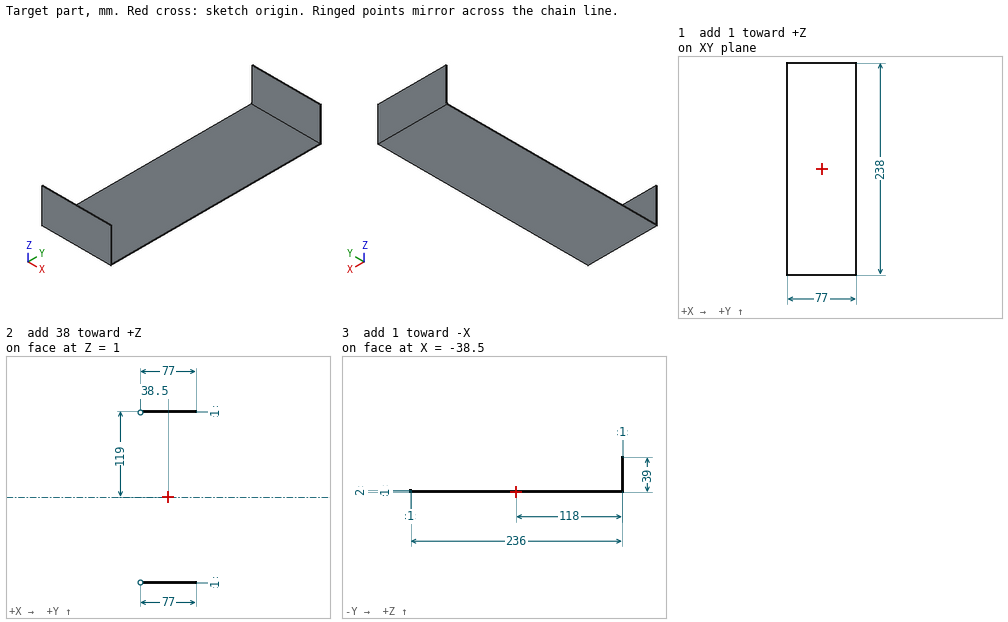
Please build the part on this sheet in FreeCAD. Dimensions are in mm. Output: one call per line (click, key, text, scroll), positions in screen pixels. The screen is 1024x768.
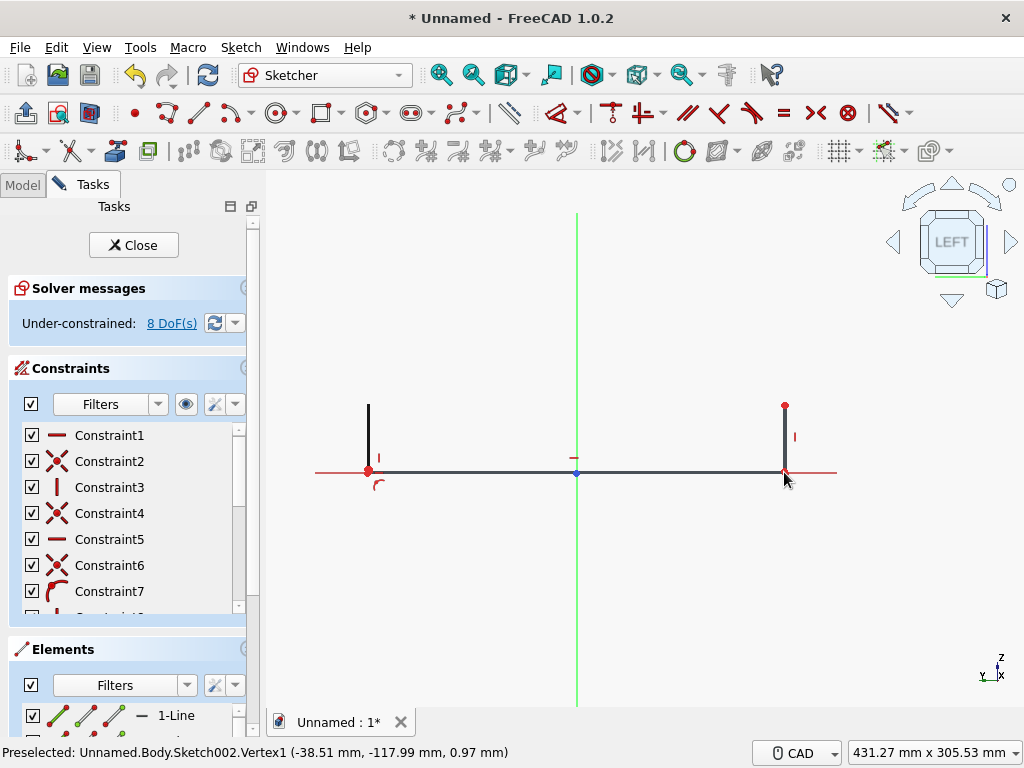
scroll(785, 406, up, 14)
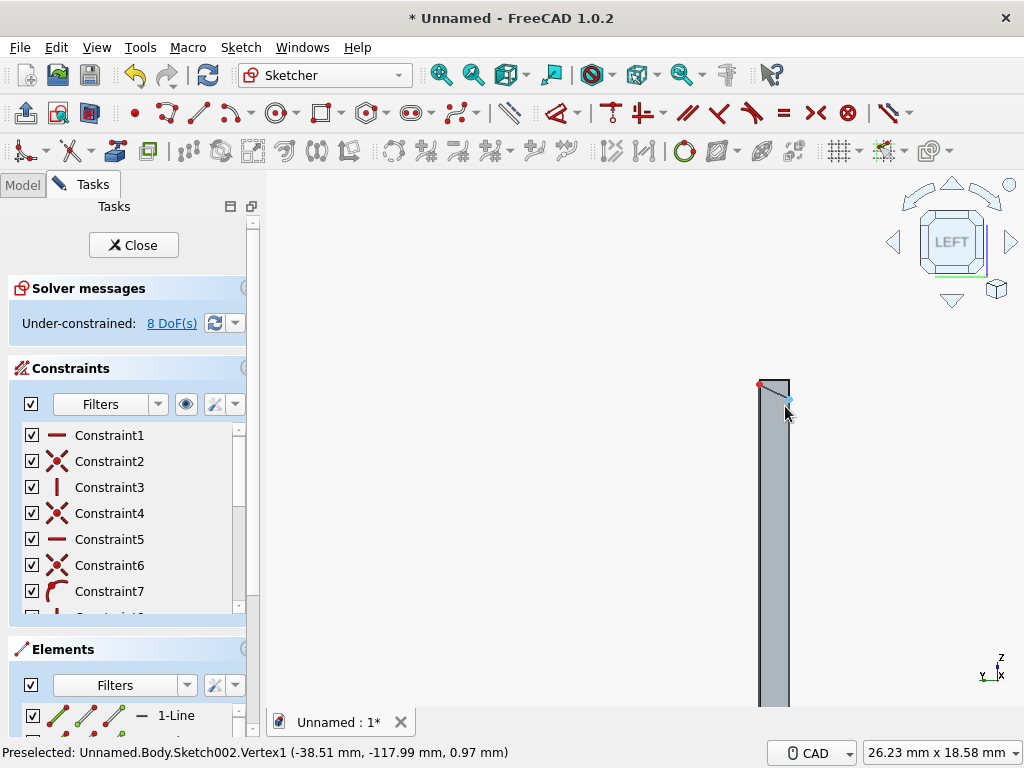
click(774, 392)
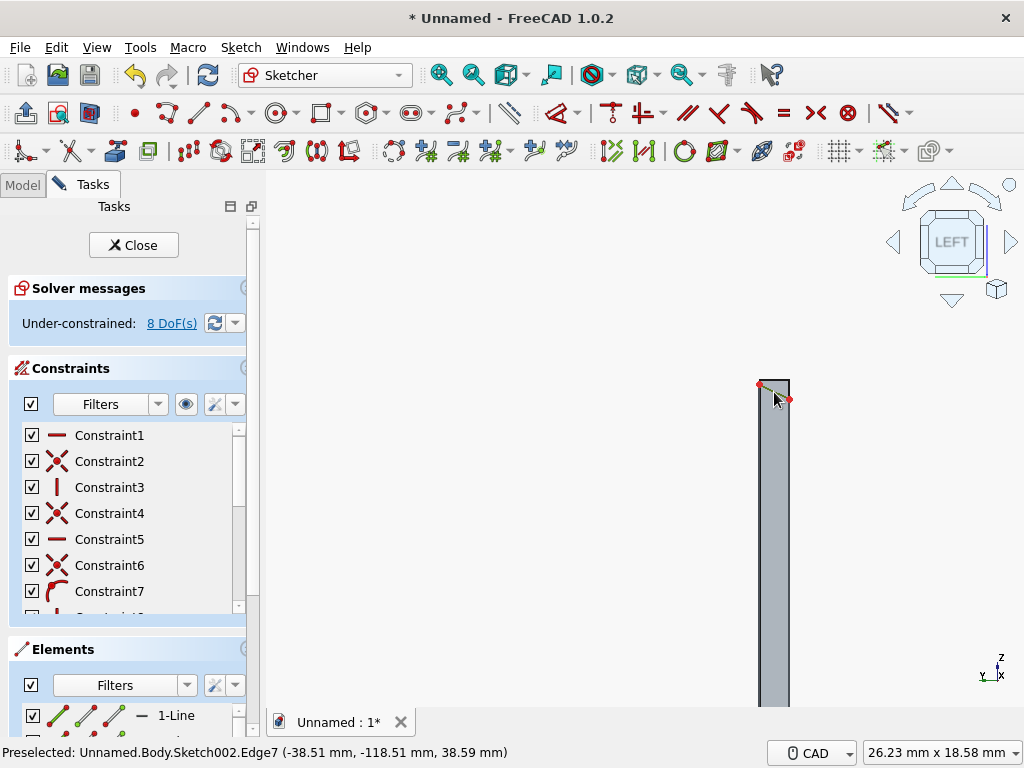
key(h)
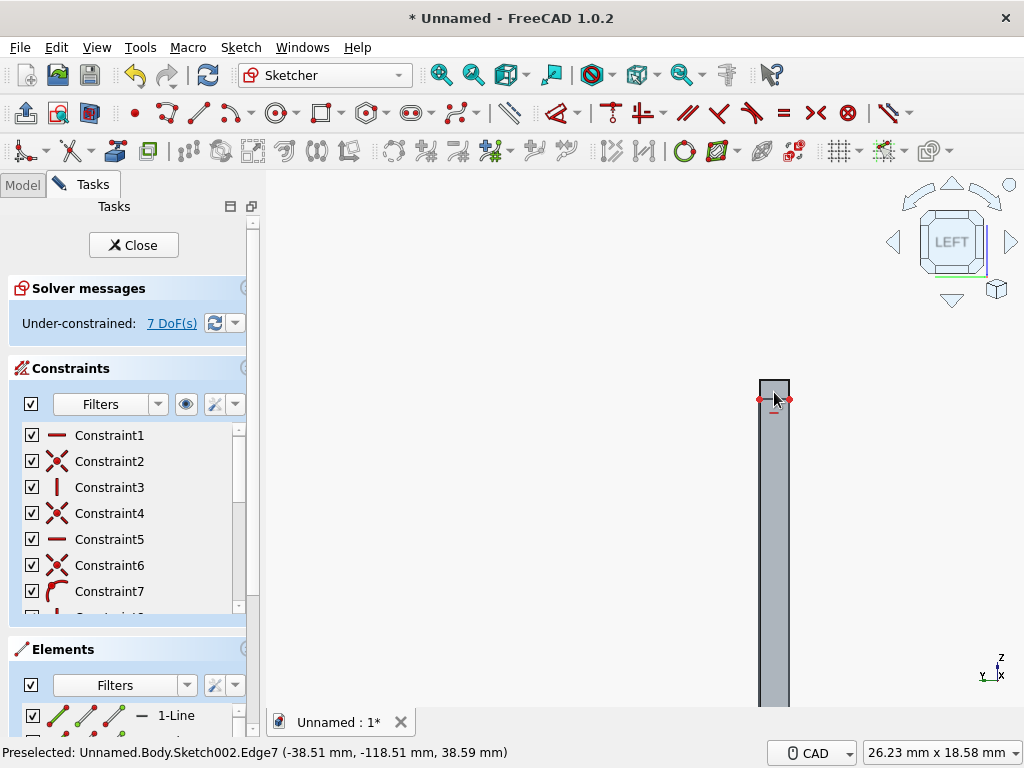
click(556, 114)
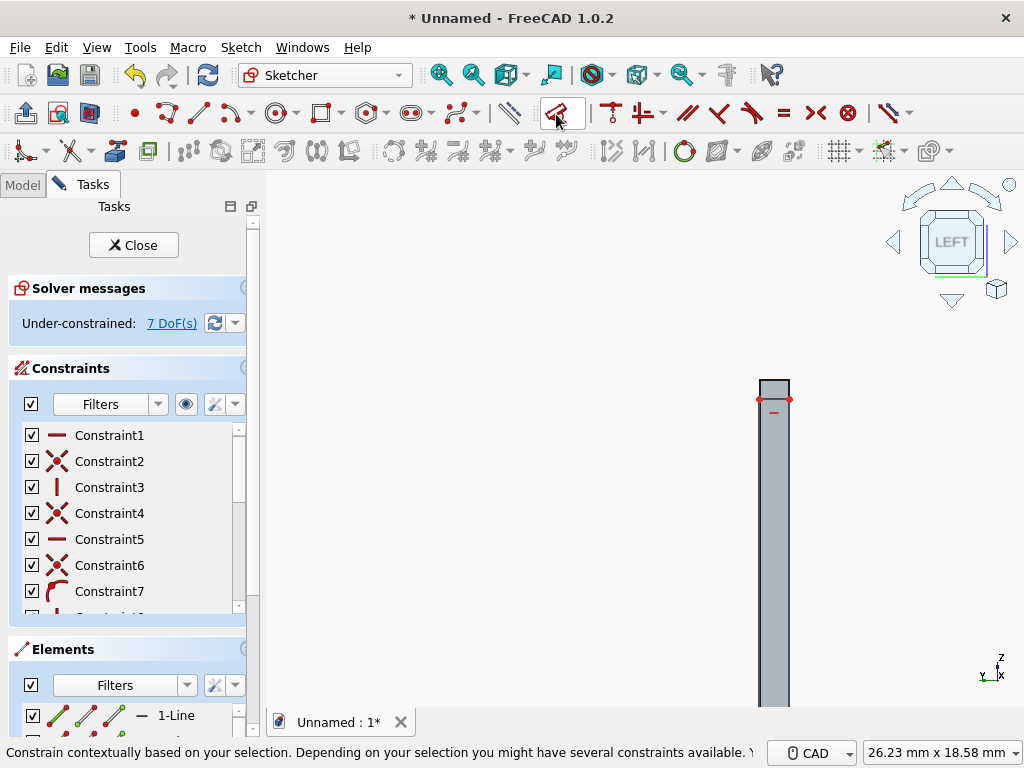
scroll(785, 406, down, 14)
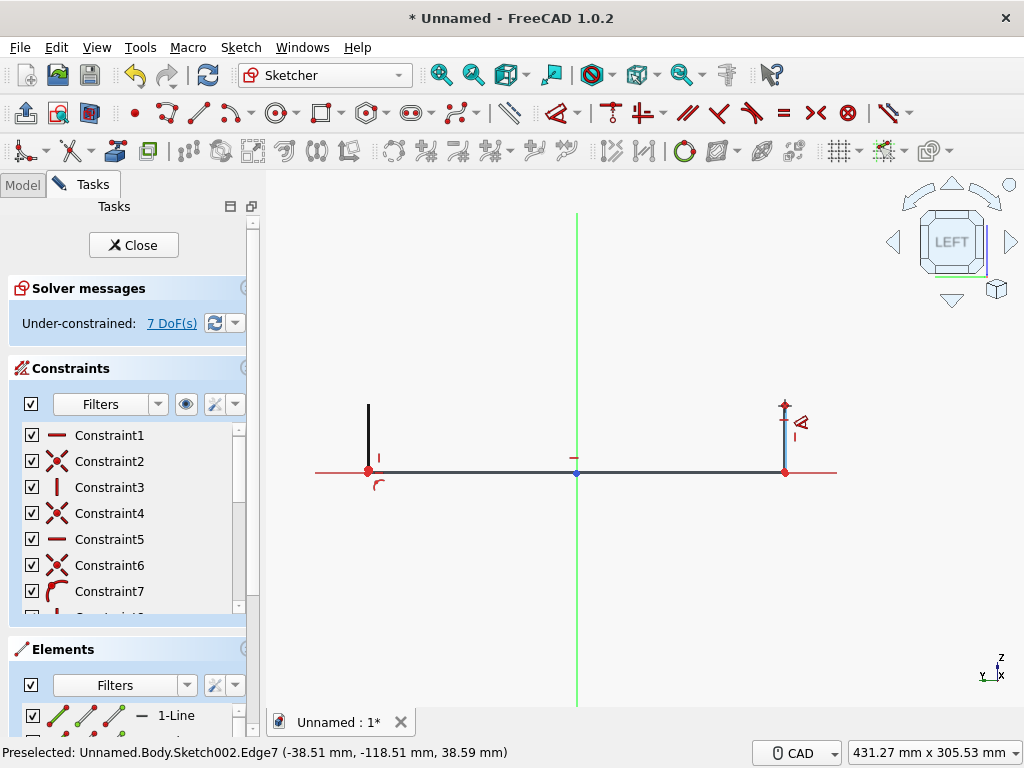
scroll(369, 471, up, 16)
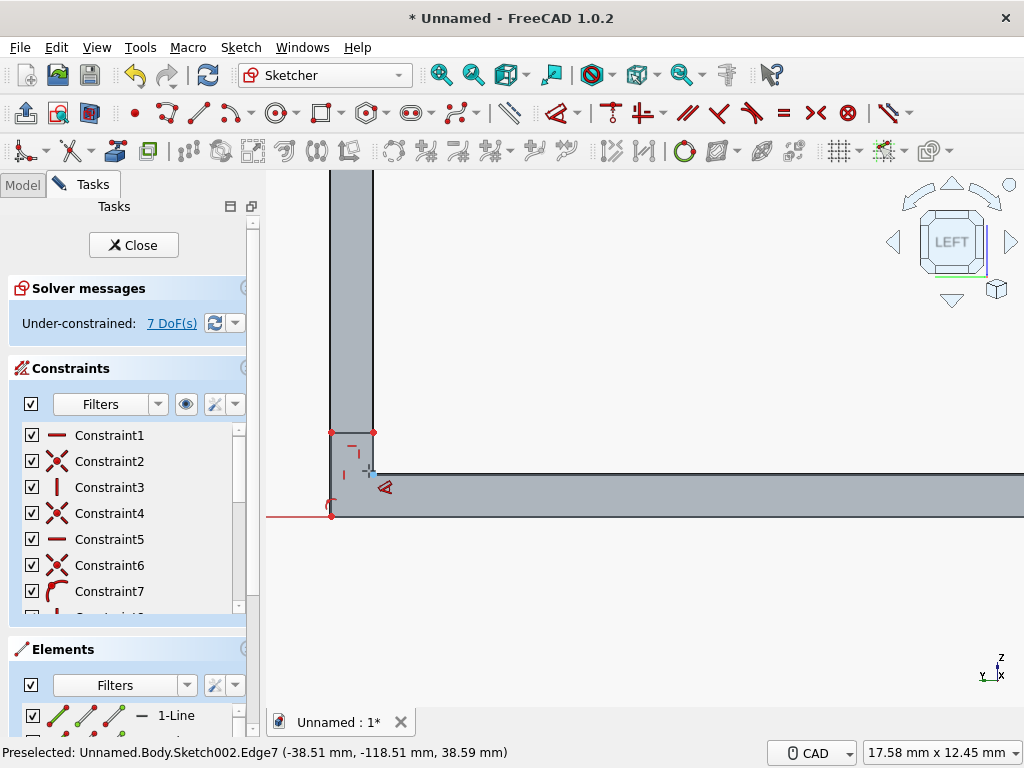
click(373, 458)
click(407, 454)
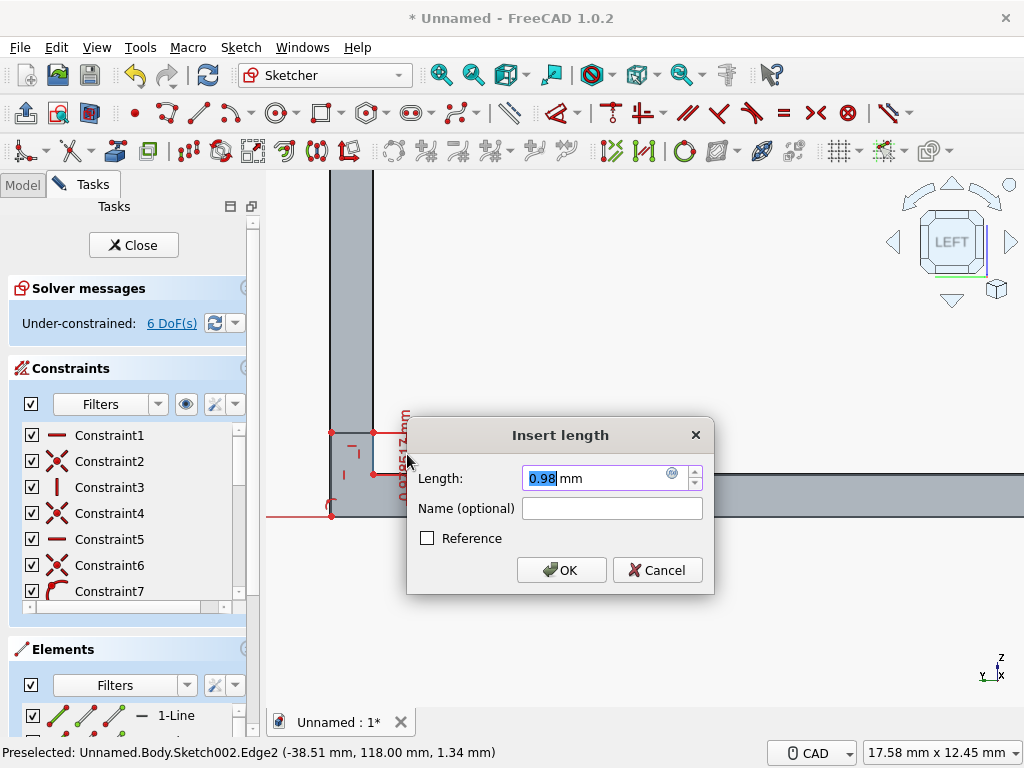
text(1)
key(Return)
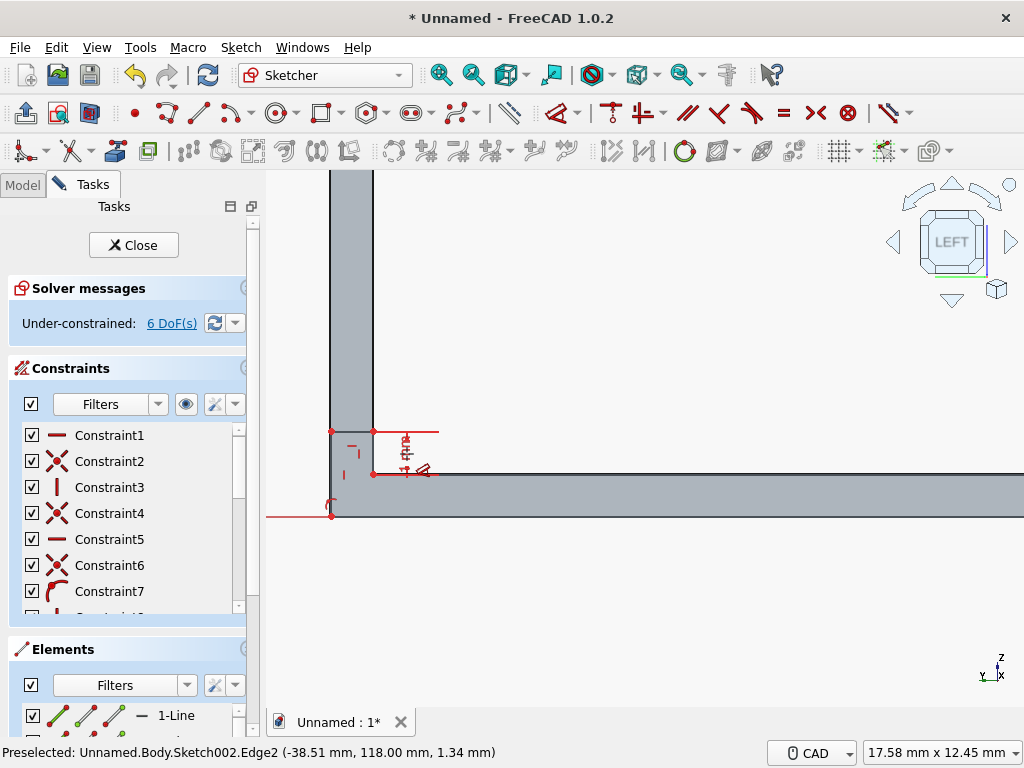
click(361, 432)
click(352, 398)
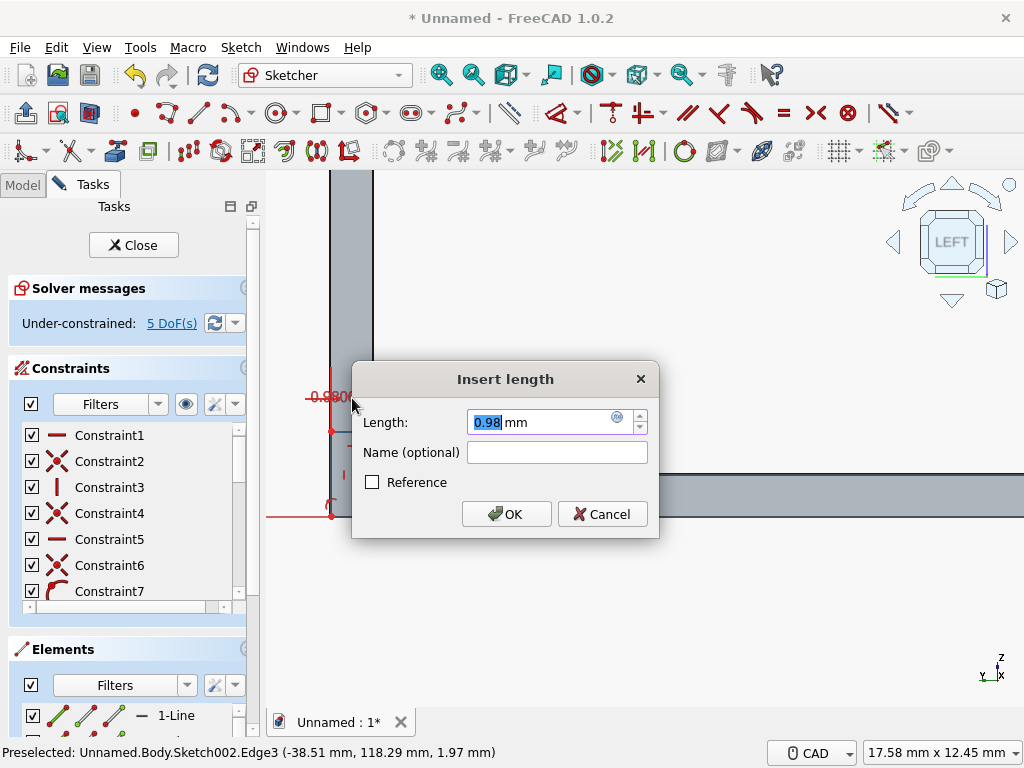
text(1)
key(Return)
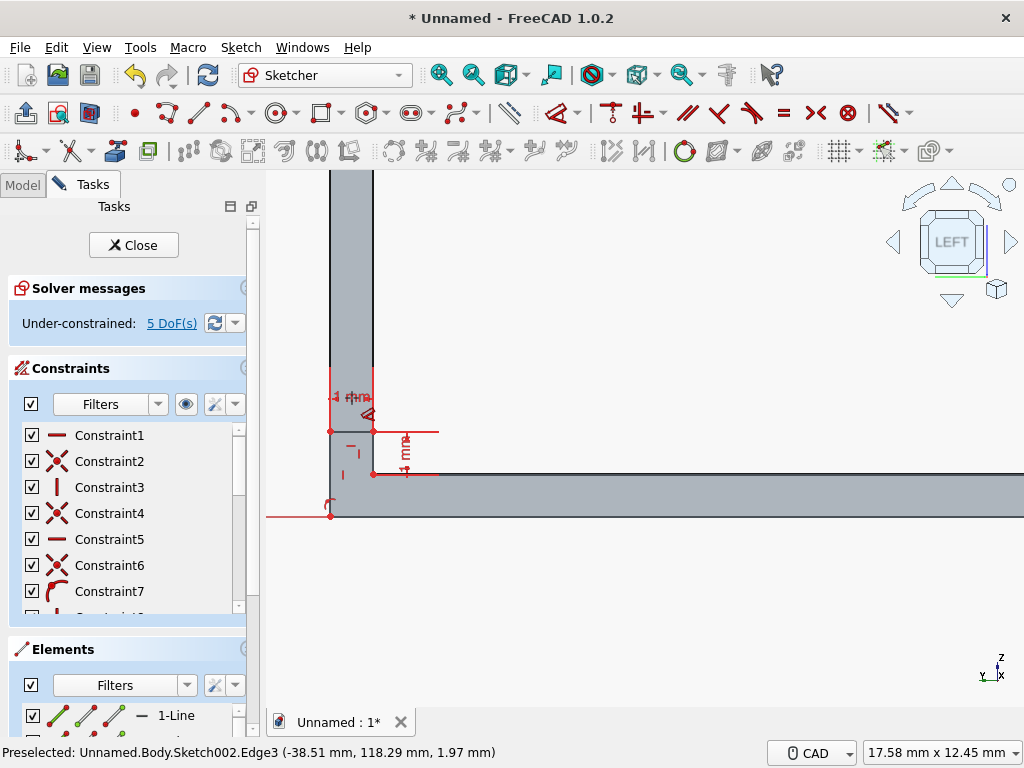
click(330, 457)
click(296, 474)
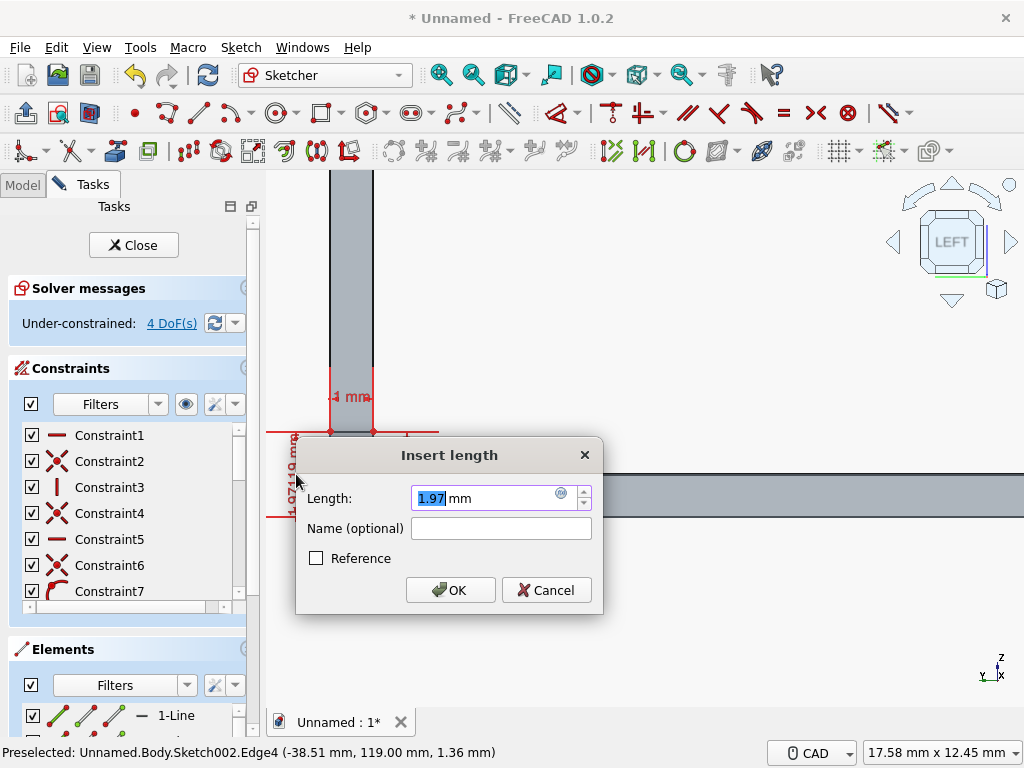
text(2)
key(Return)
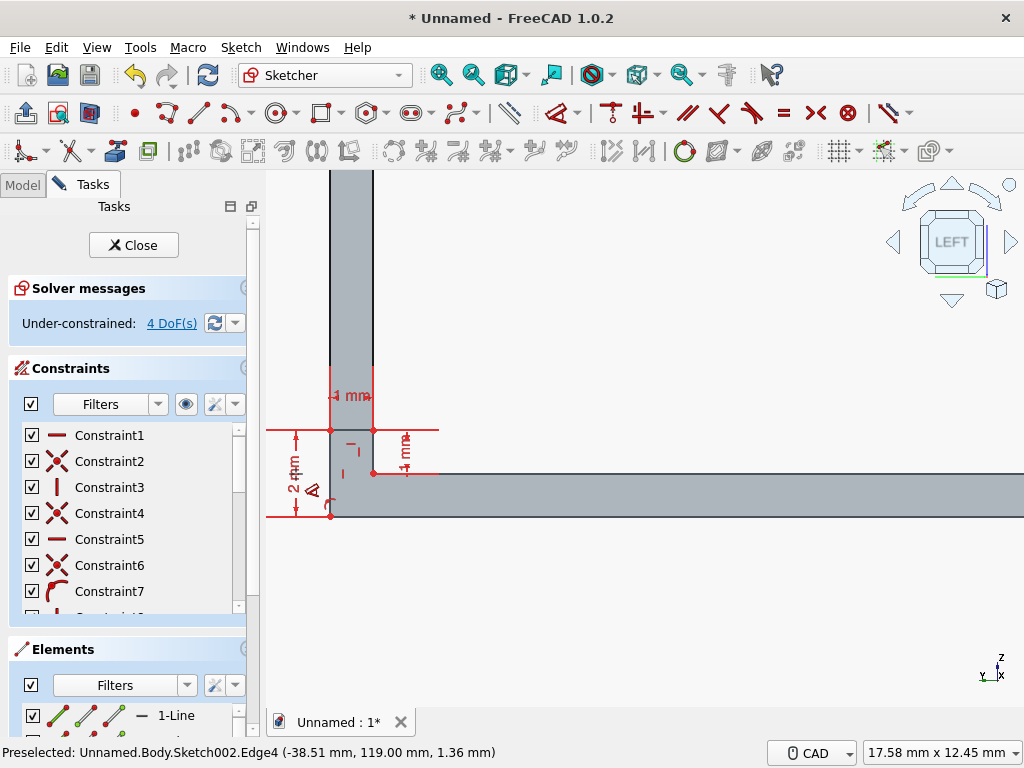
scroll(321, 478, down, 15)